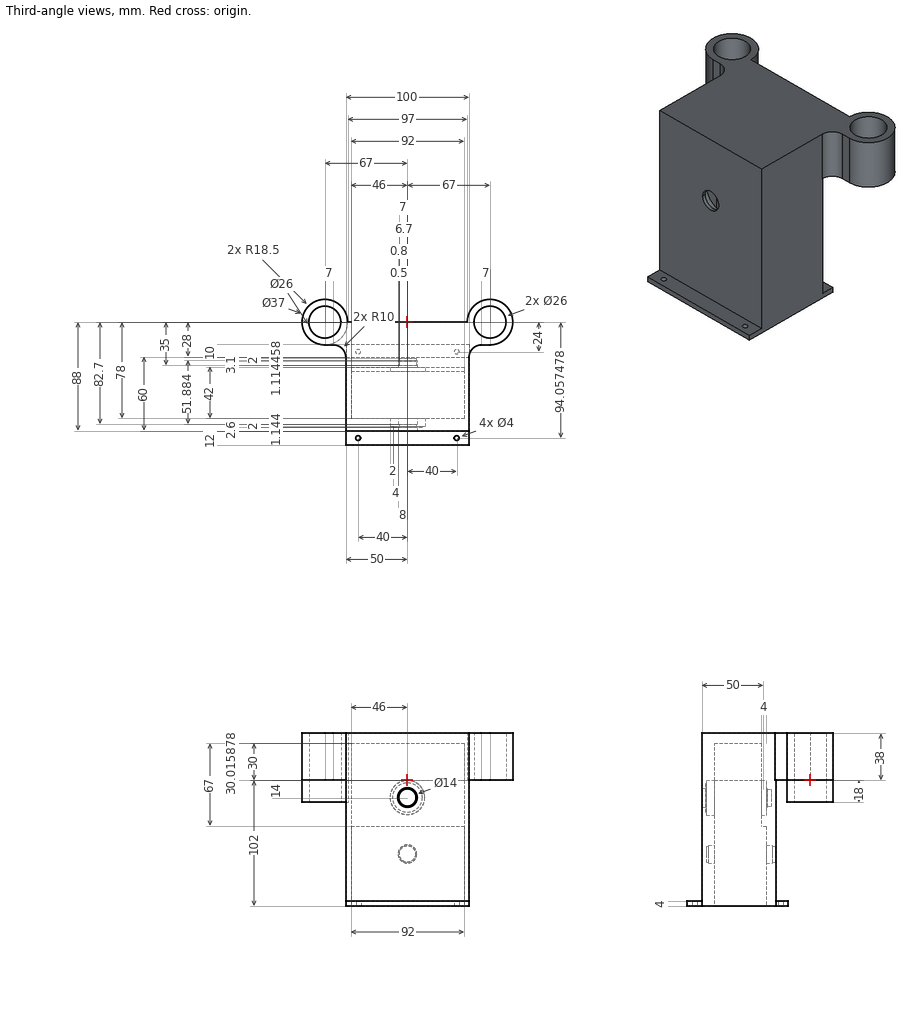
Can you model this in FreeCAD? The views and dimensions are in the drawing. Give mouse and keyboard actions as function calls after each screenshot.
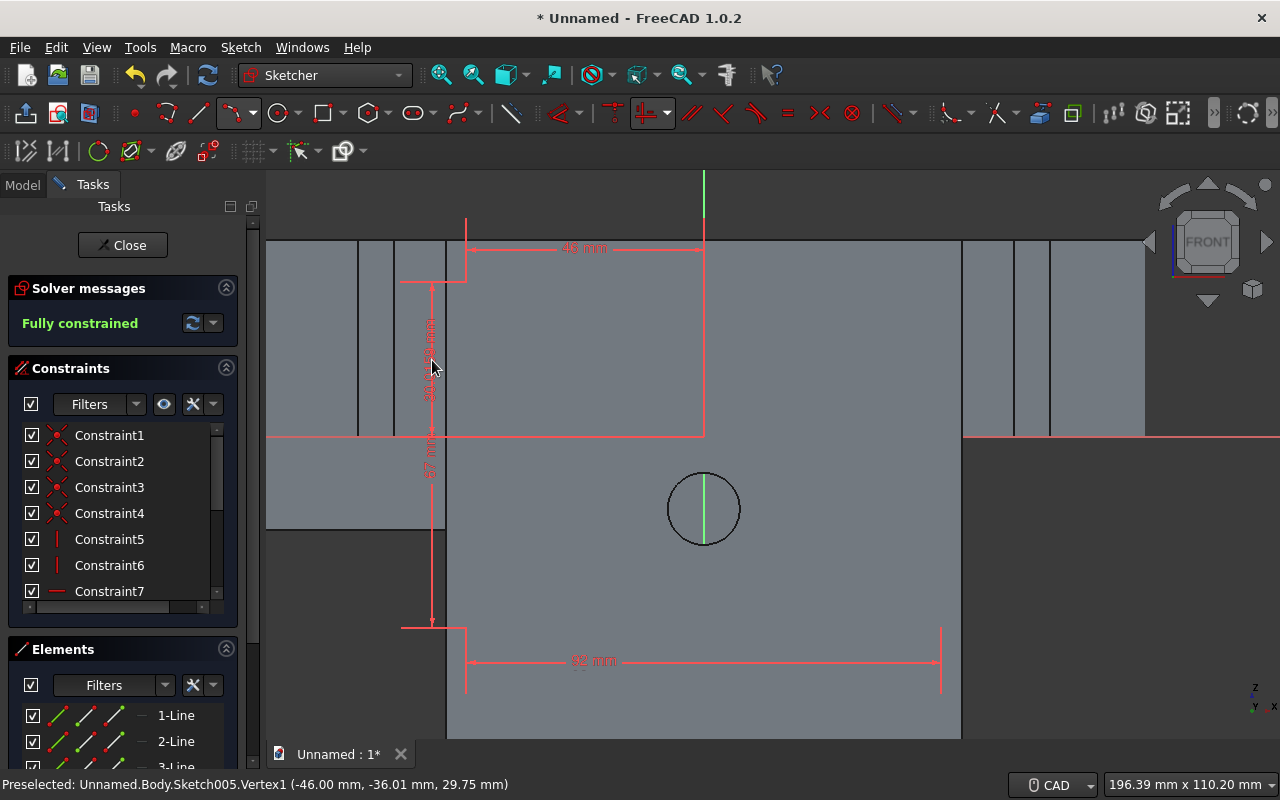
click(123, 245)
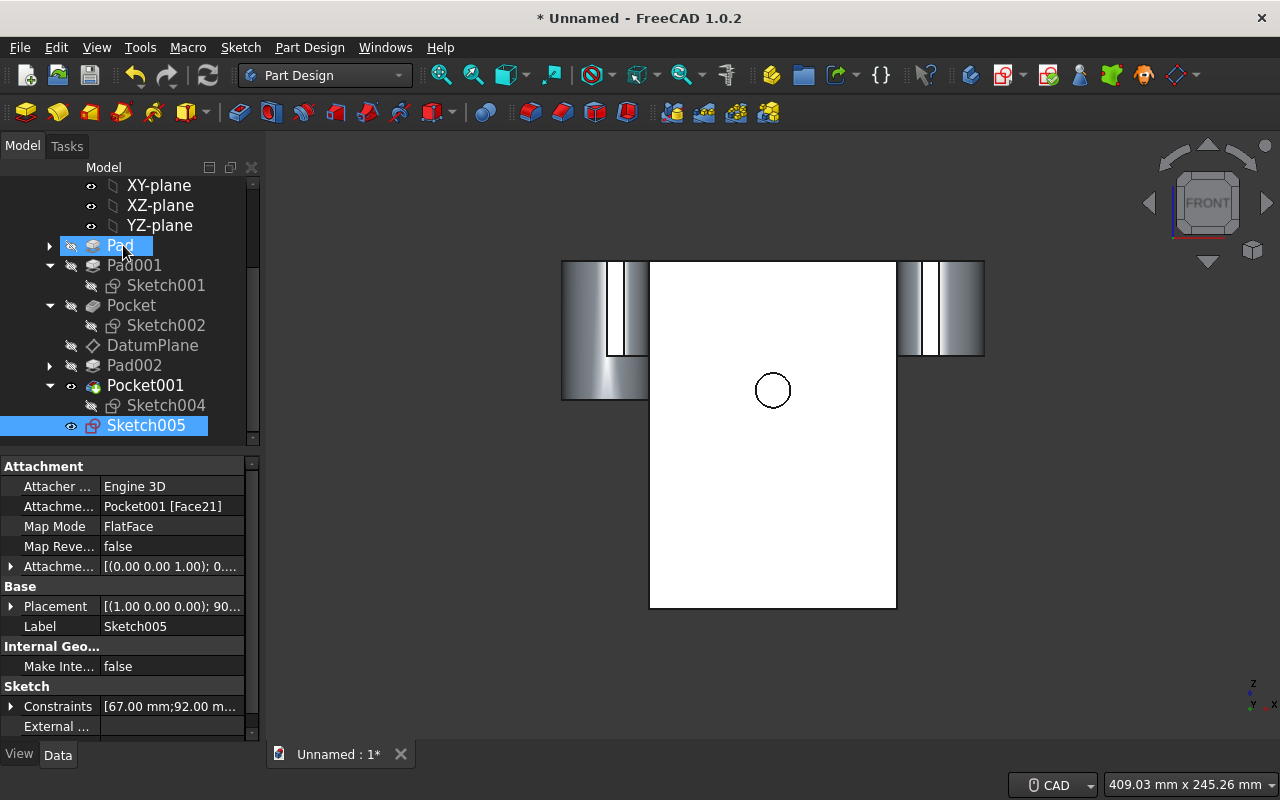
click(26, 112)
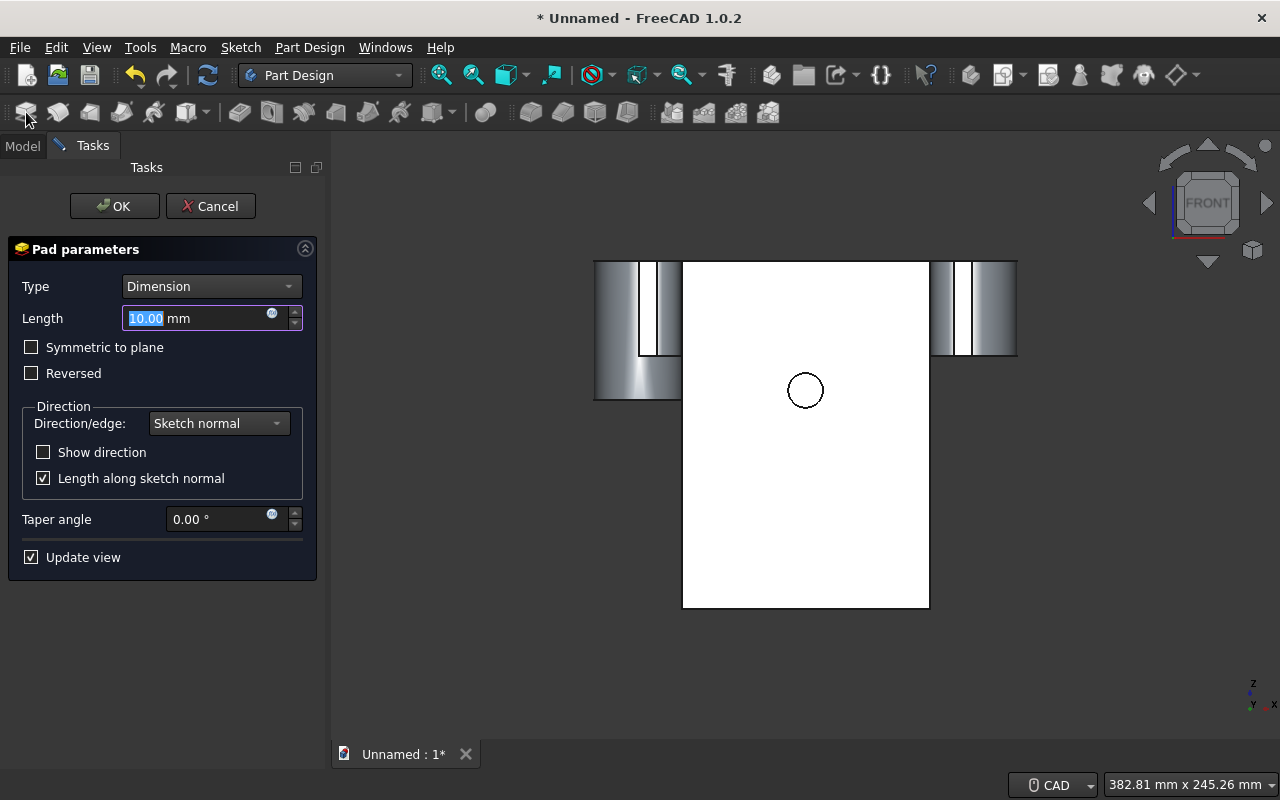
text(4)
key(Tab)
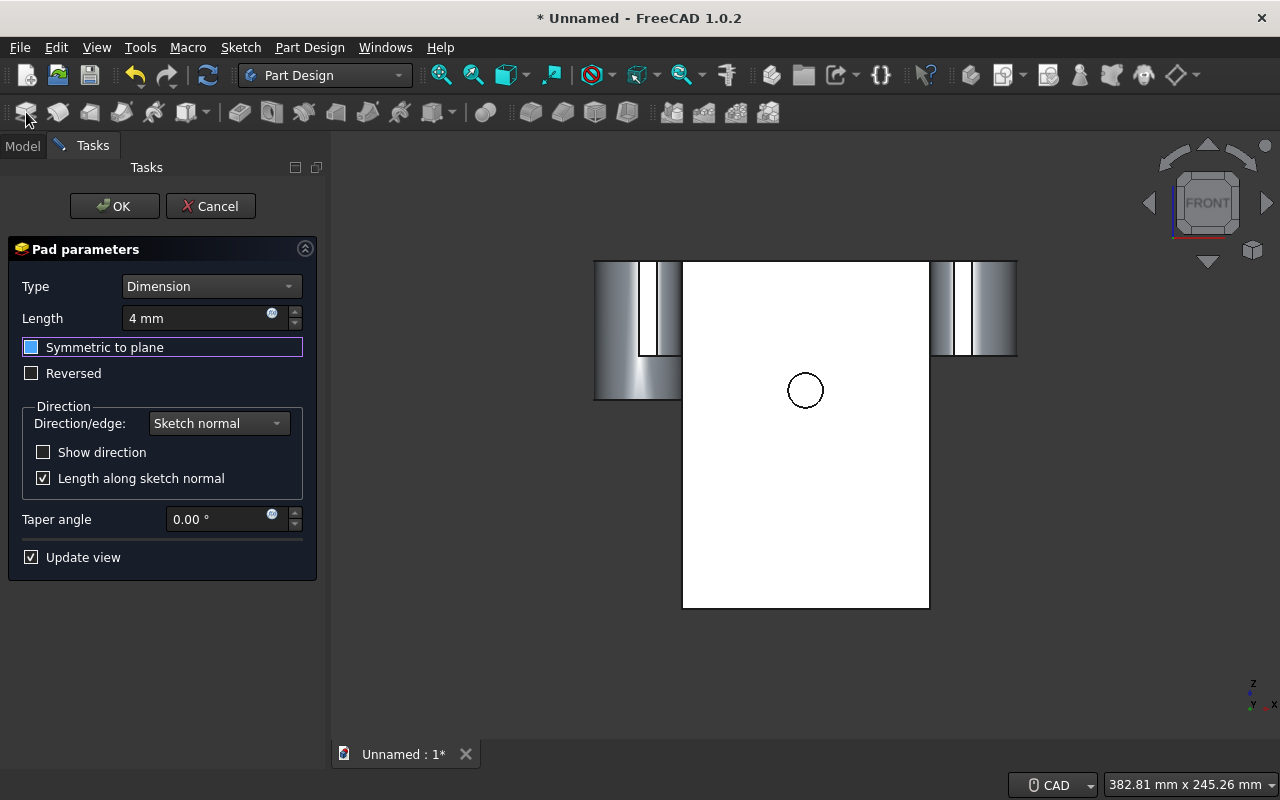
click(115, 206)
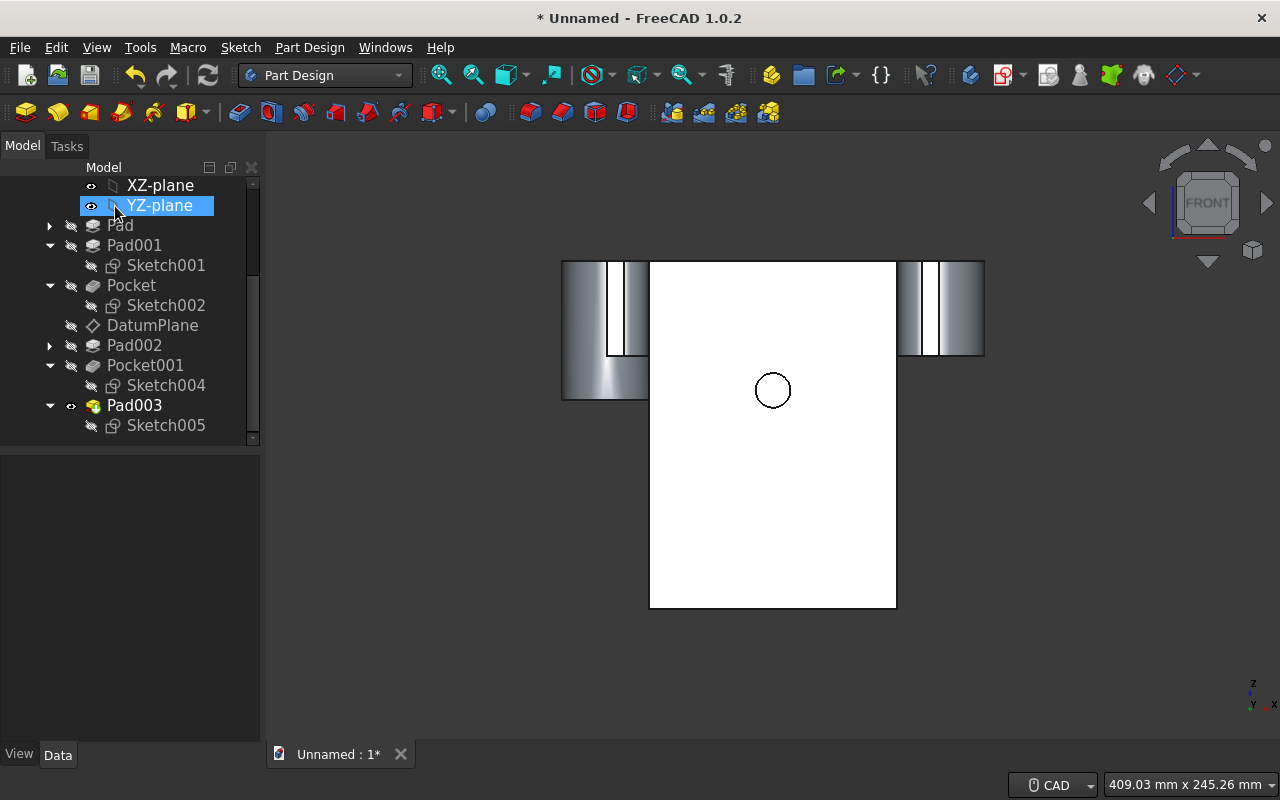
scroll(160, 301, down, 3)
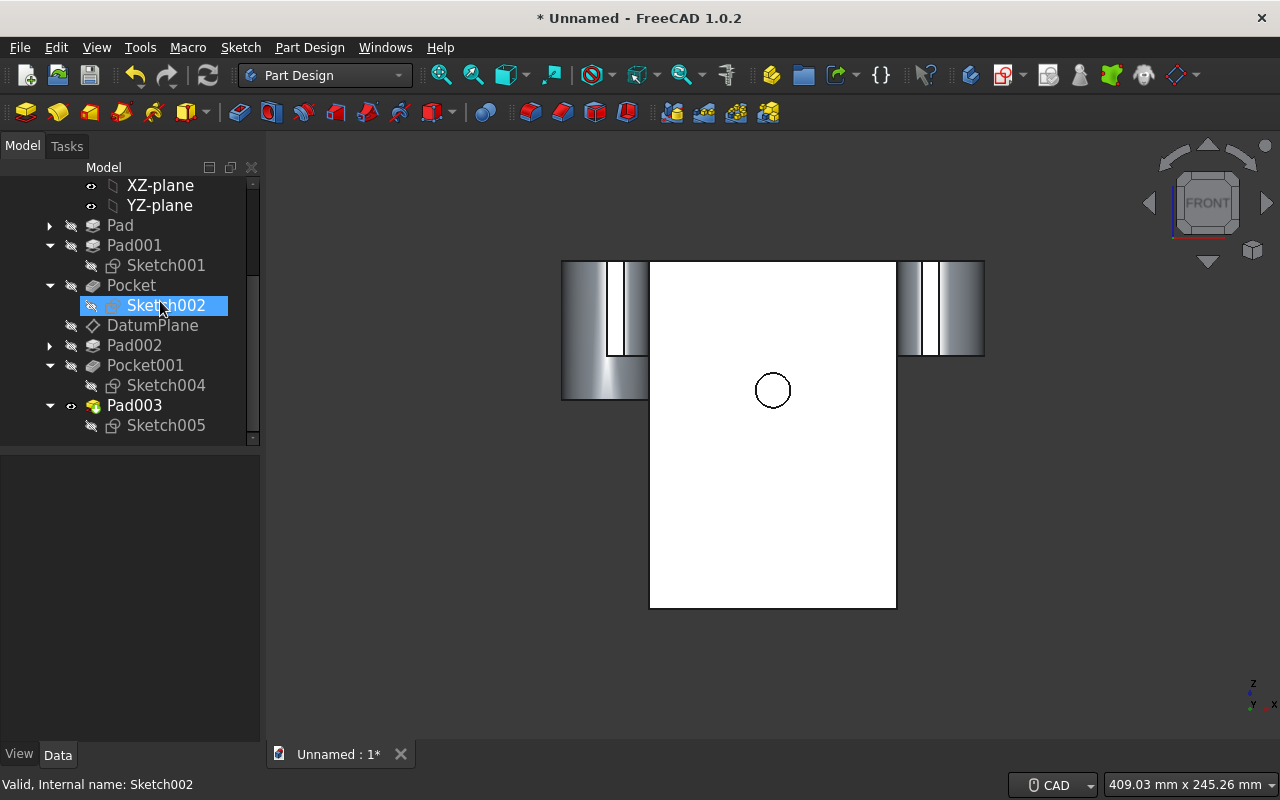
scroll(160, 301, up, 15)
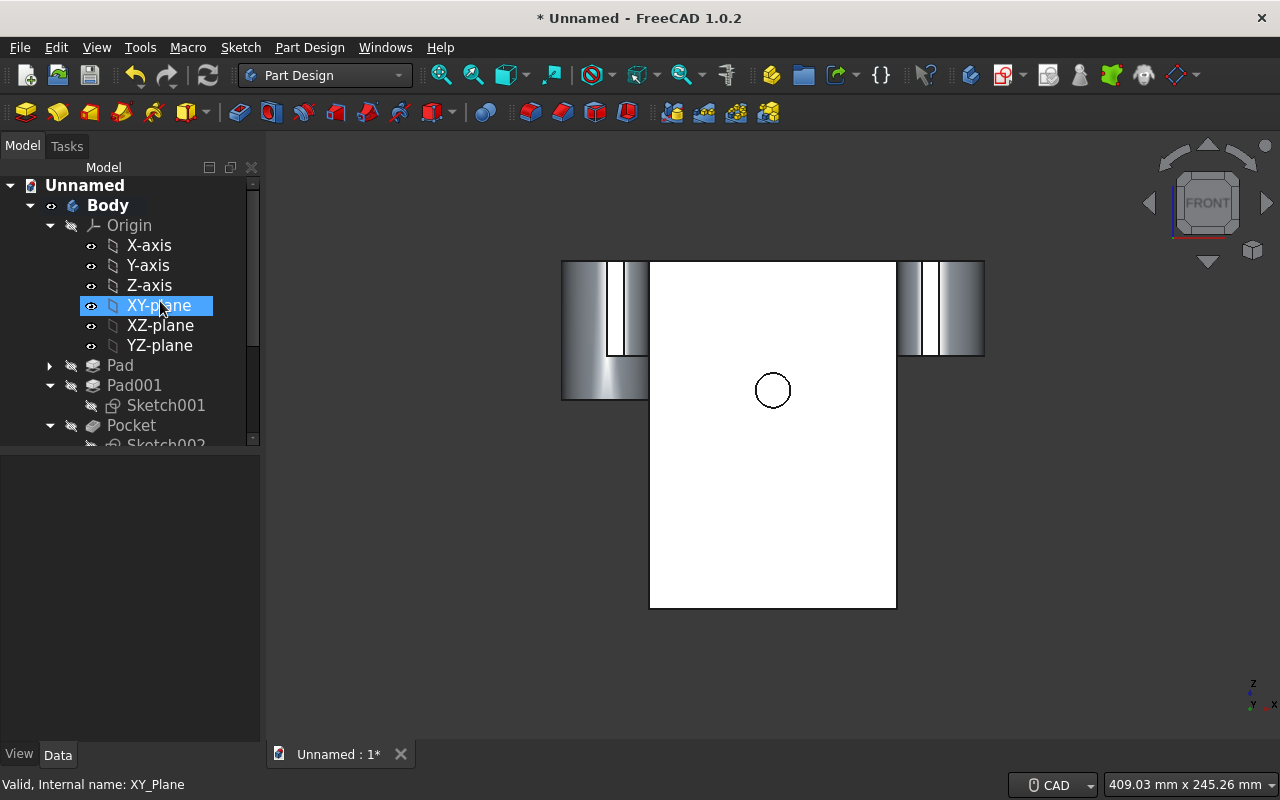
click(136, 306)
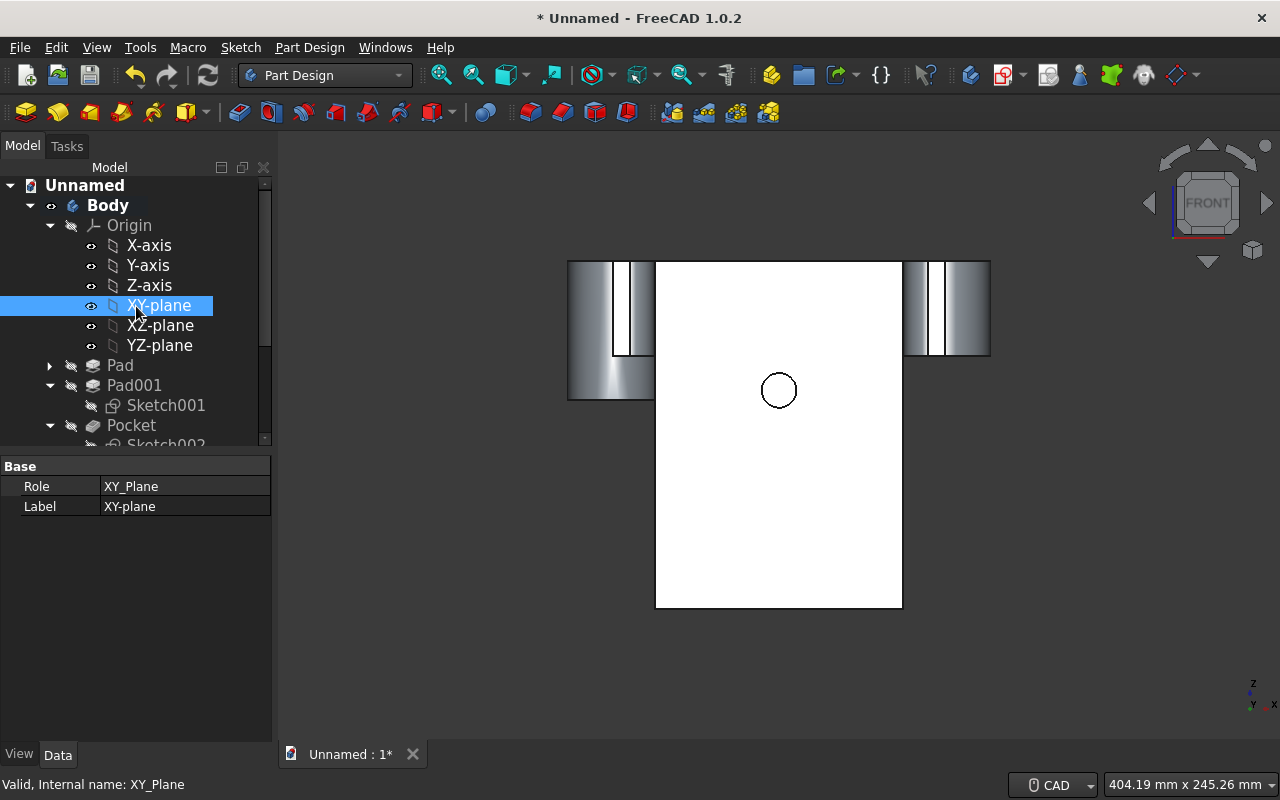
click(1176, 76)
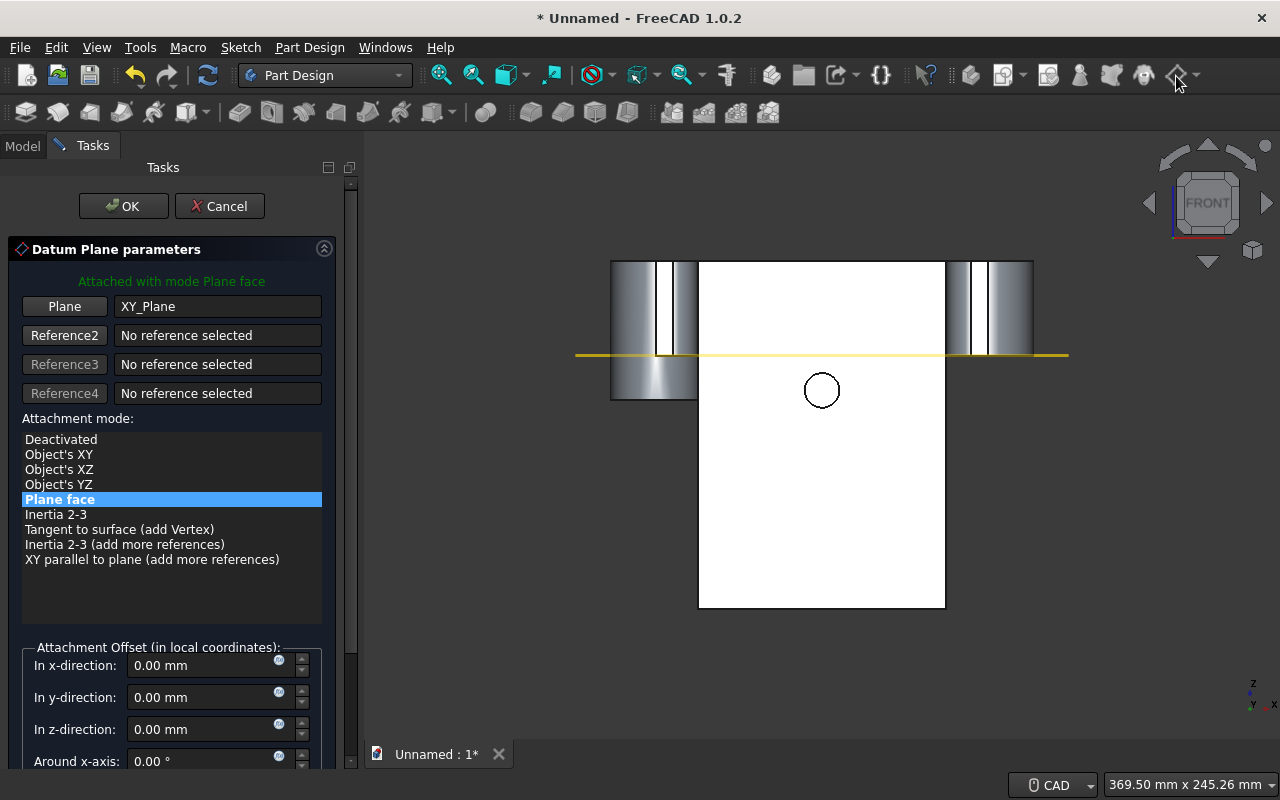
triple_click(210, 729)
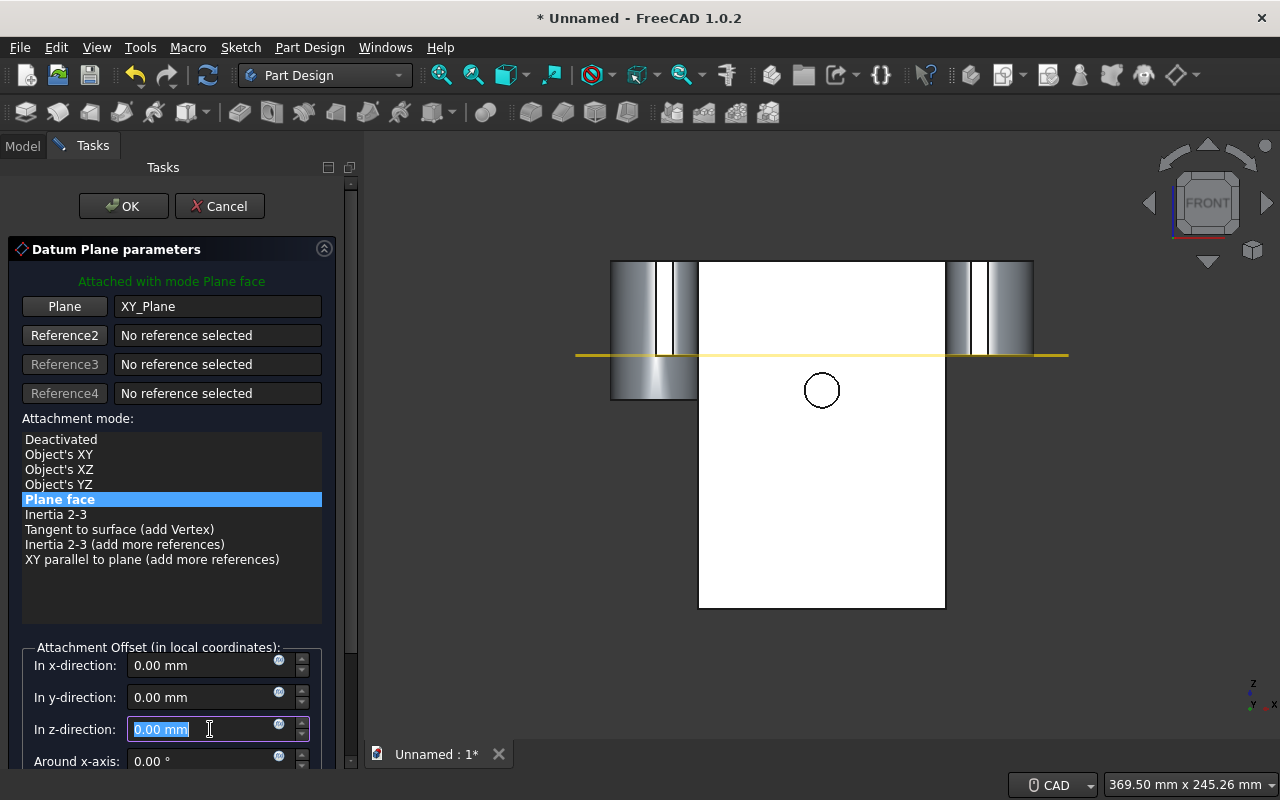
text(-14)
key(Tab)